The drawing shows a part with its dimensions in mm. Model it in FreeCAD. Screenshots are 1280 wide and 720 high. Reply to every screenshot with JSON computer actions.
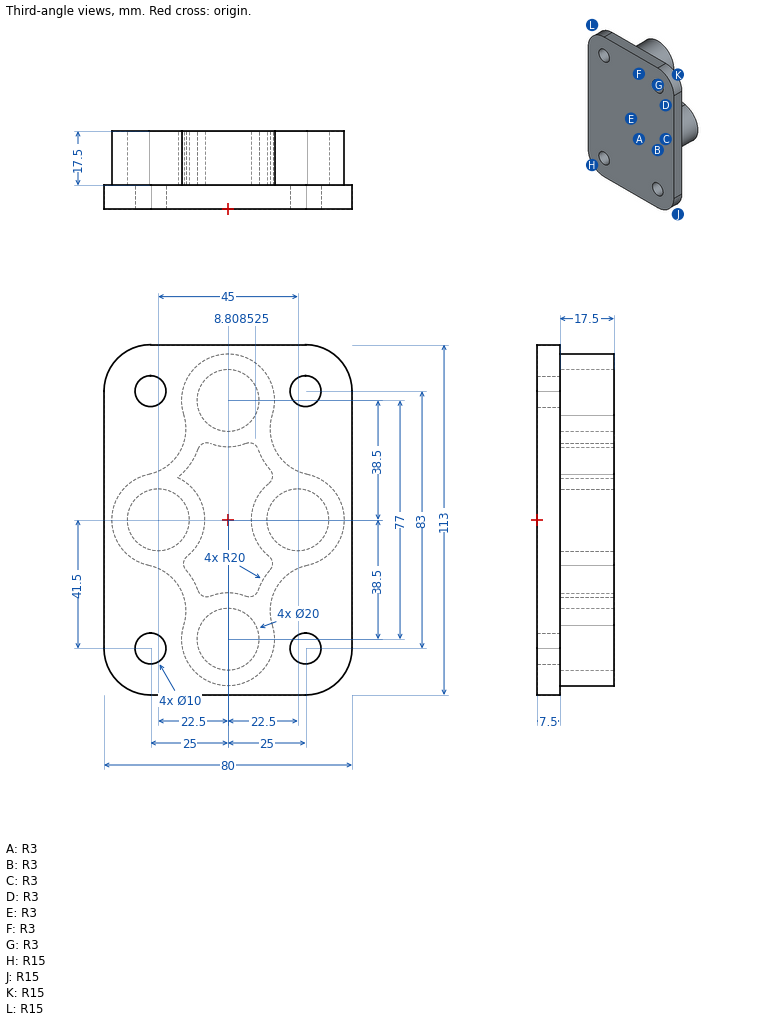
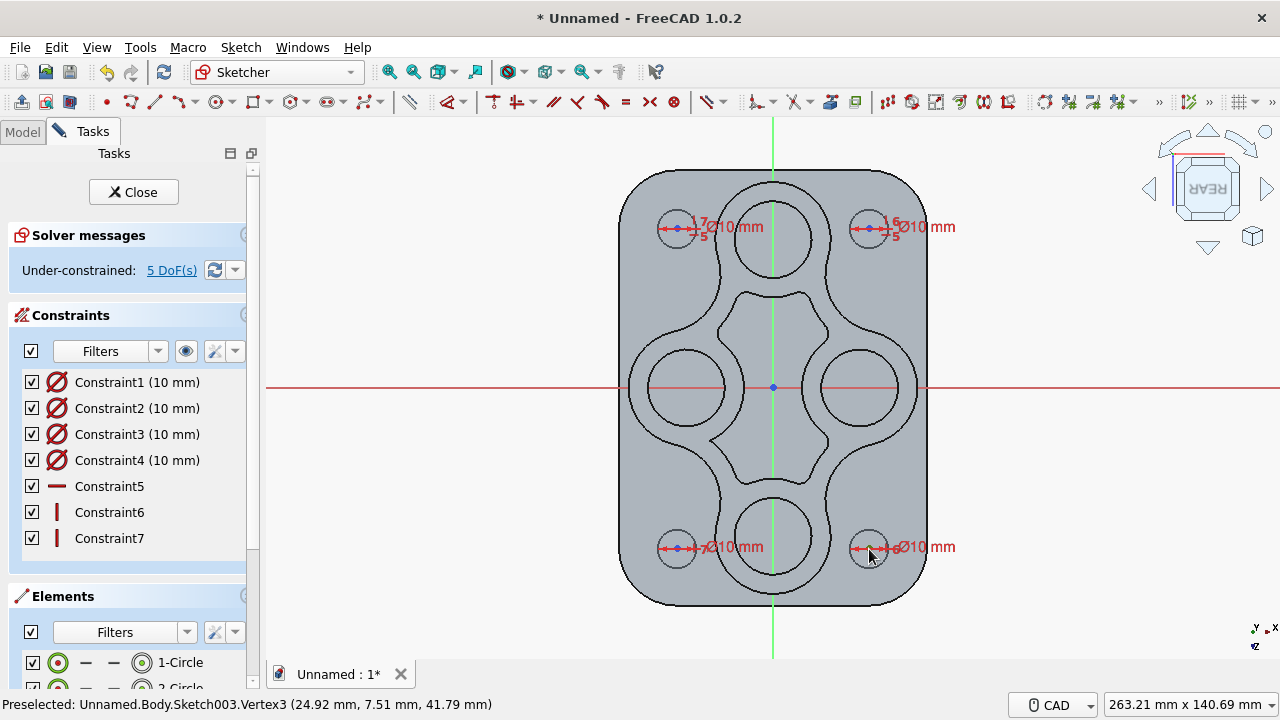
{"action": "left_click", "coordinate": [677, 549]}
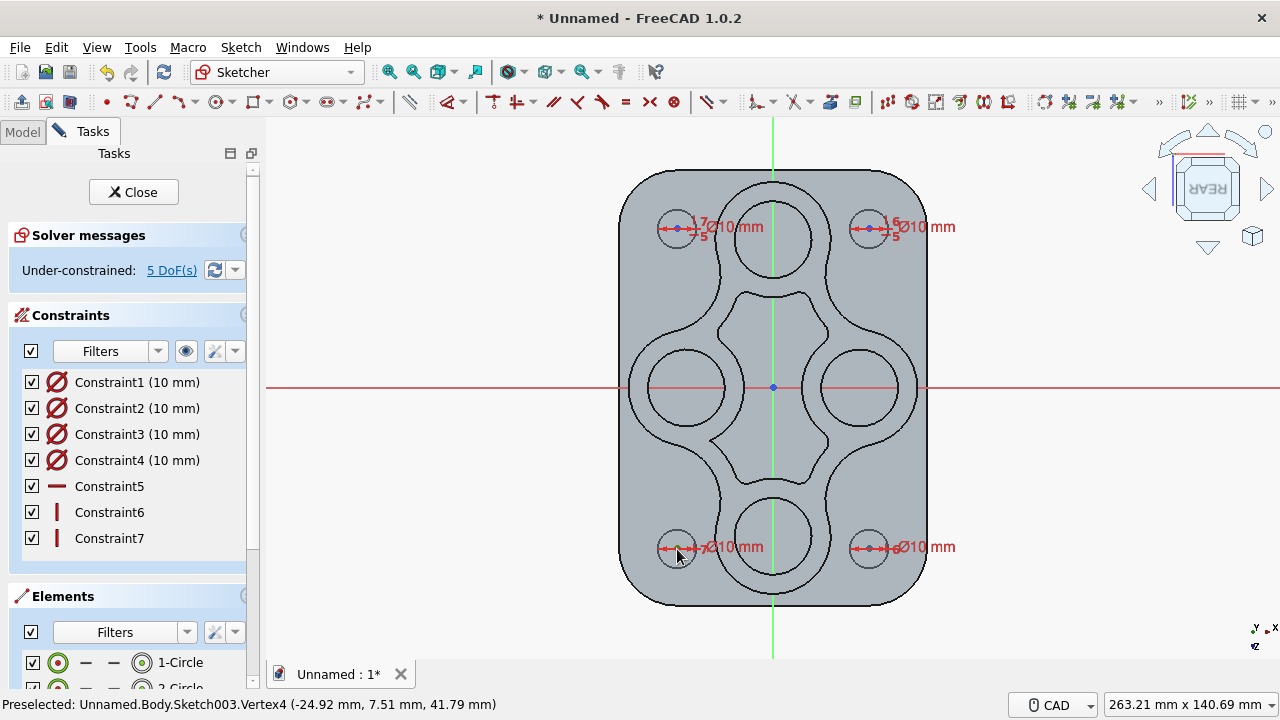
{"action": "left_click", "coordinate": [536, 102]}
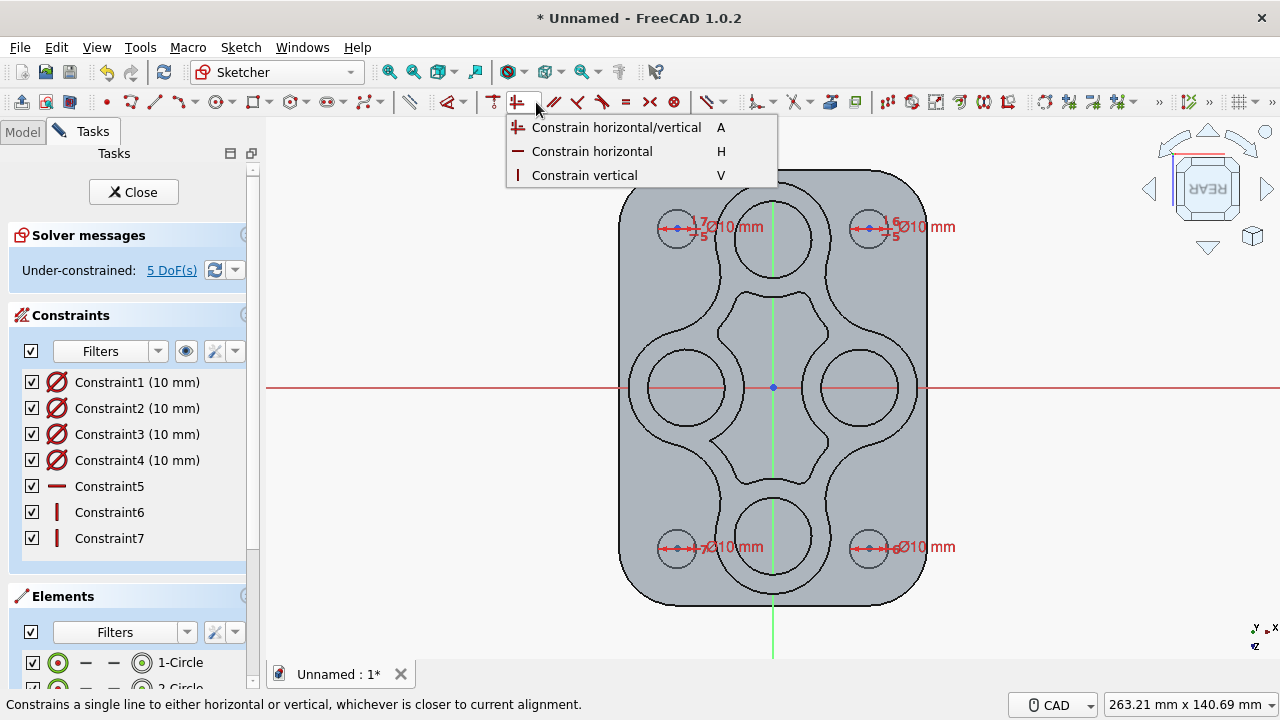
{"action": "left_click", "coordinate": [642, 151]}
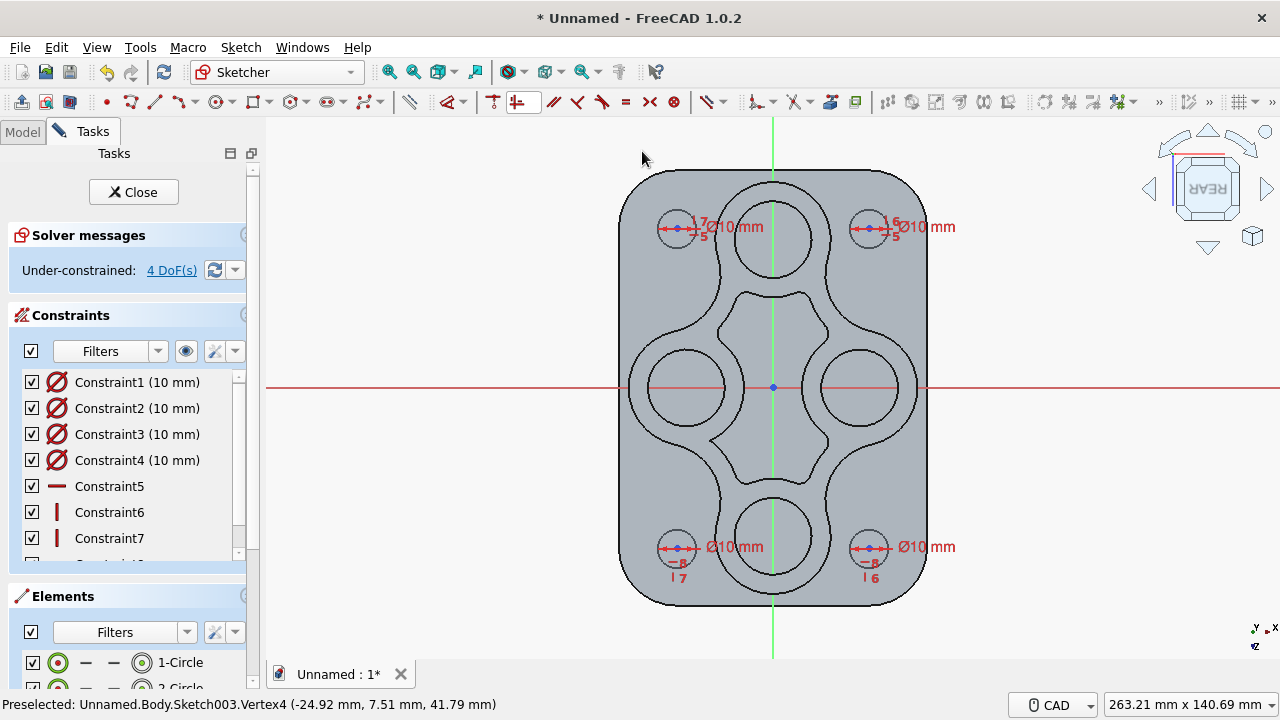
{"action": "key", "text": "d"}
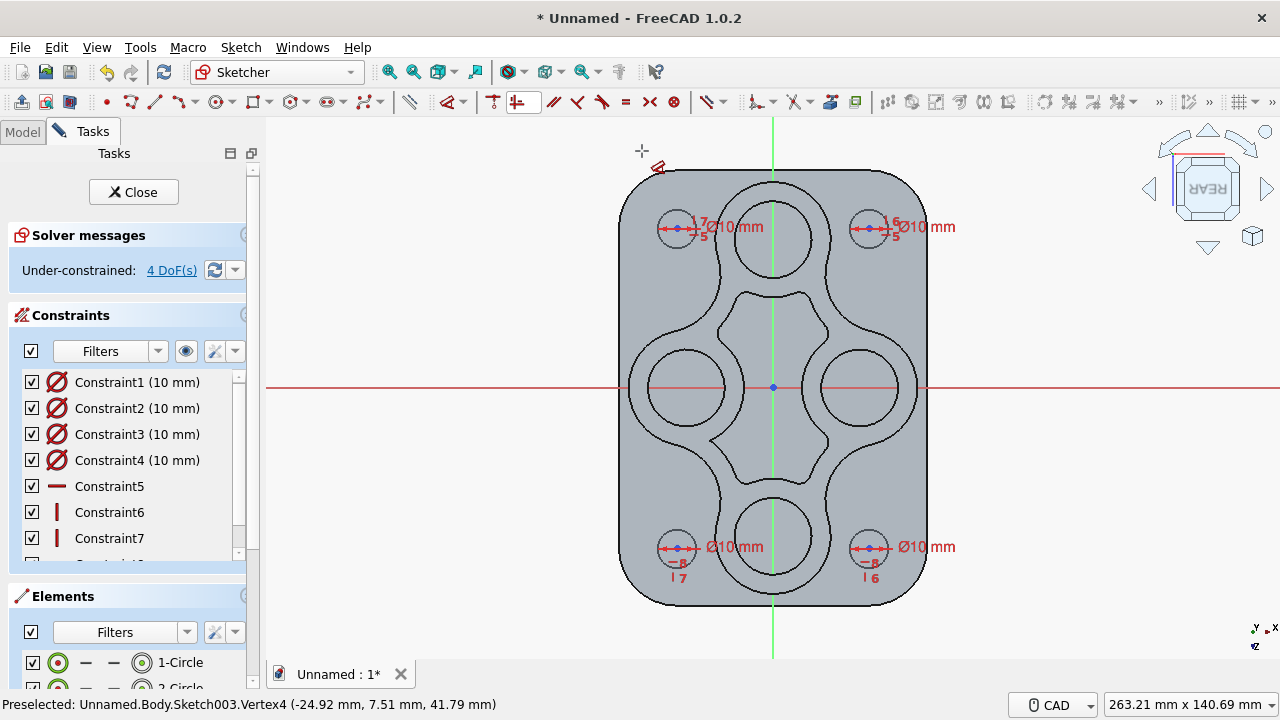
{"action": "left_click", "coordinate": [677, 229]}
{"action": "left_click", "coordinate": [725, 195]}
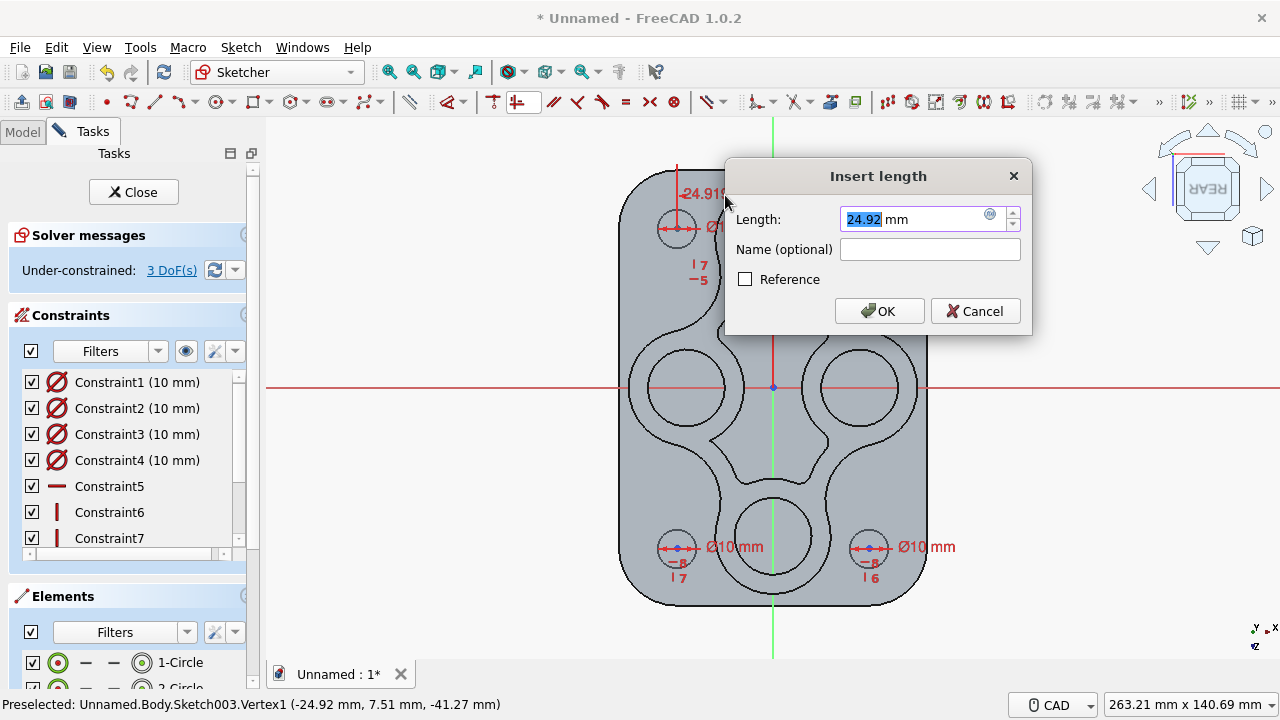
{"action": "type", "text": "25"}
{"action": "key", "text": "Return"}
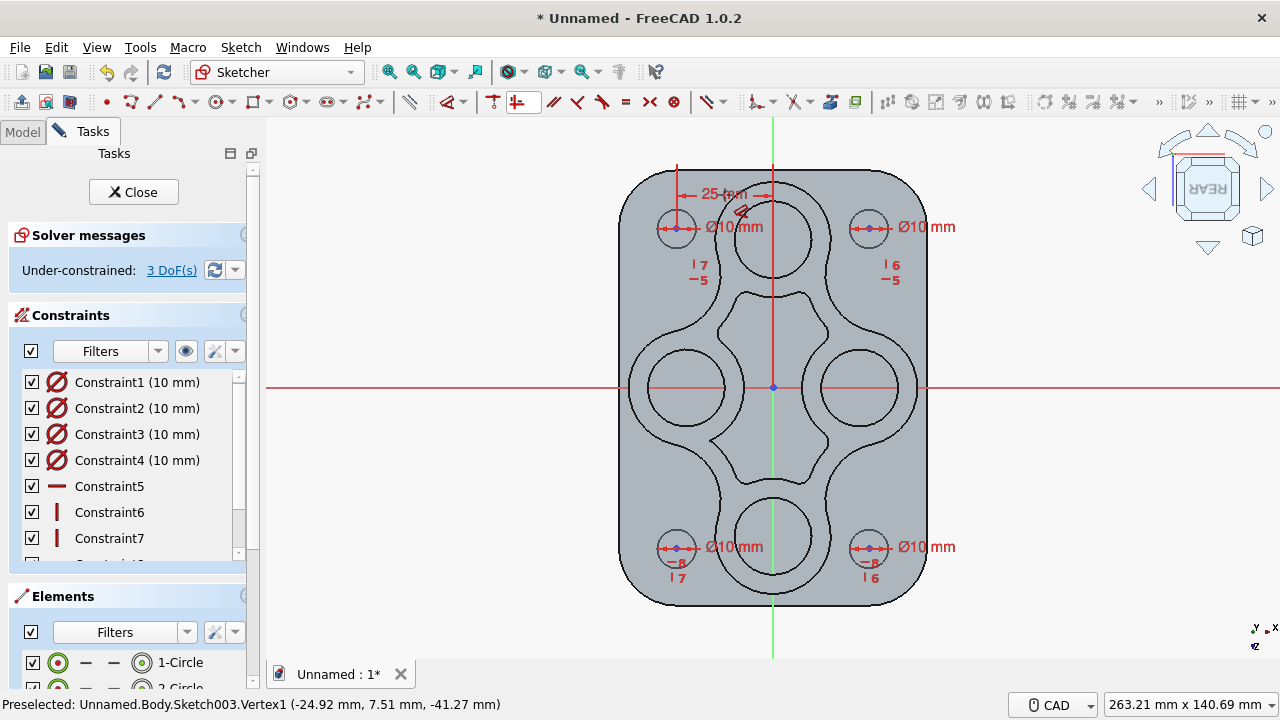
{"action": "left_click", "coordinate": [869, 229]}
{"action": "left_click", "coordinate": [821, 195]}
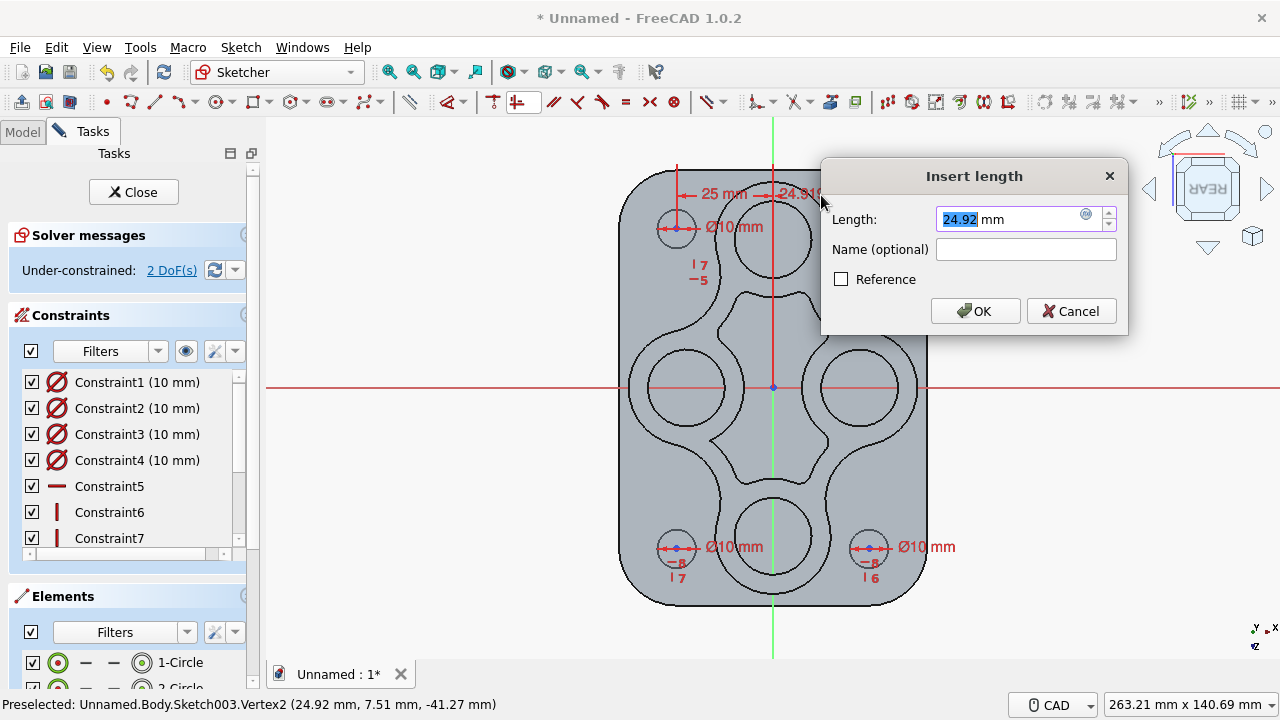
{"action": "type", "text": "25"}
{"action": "key", "text": "Return"}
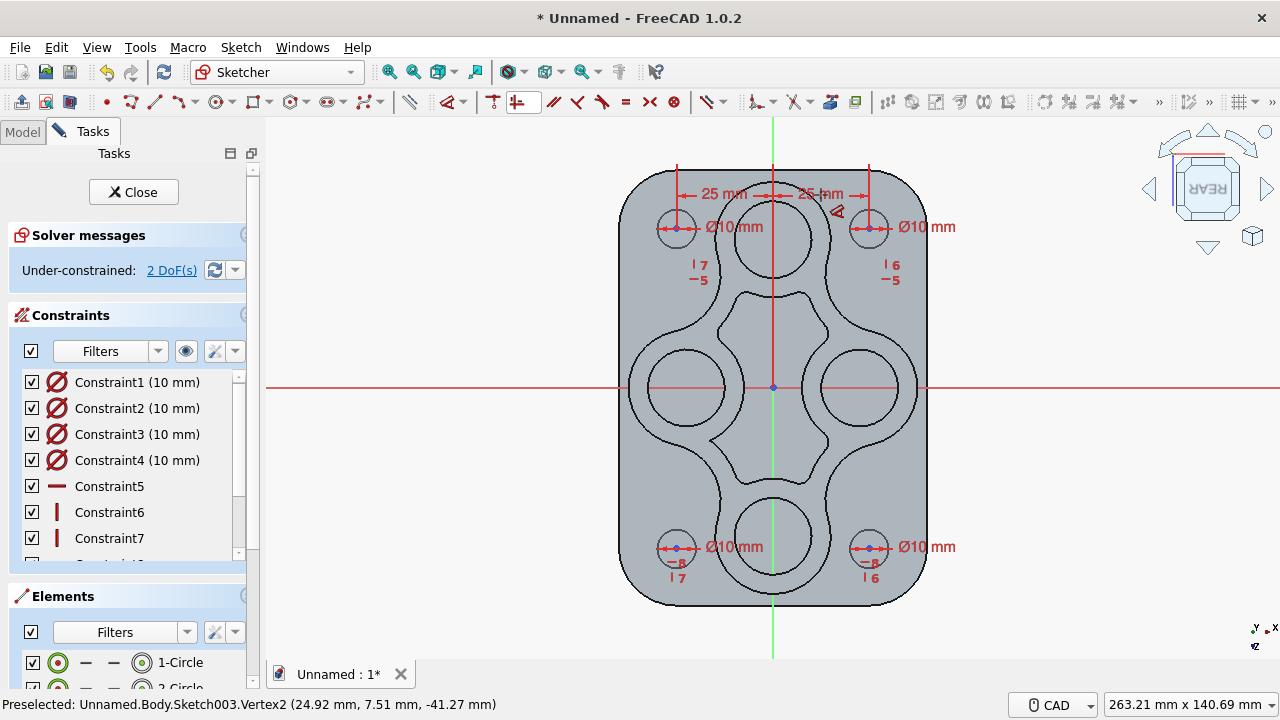
{"action": "left_click", "coordinate": [869, 229]}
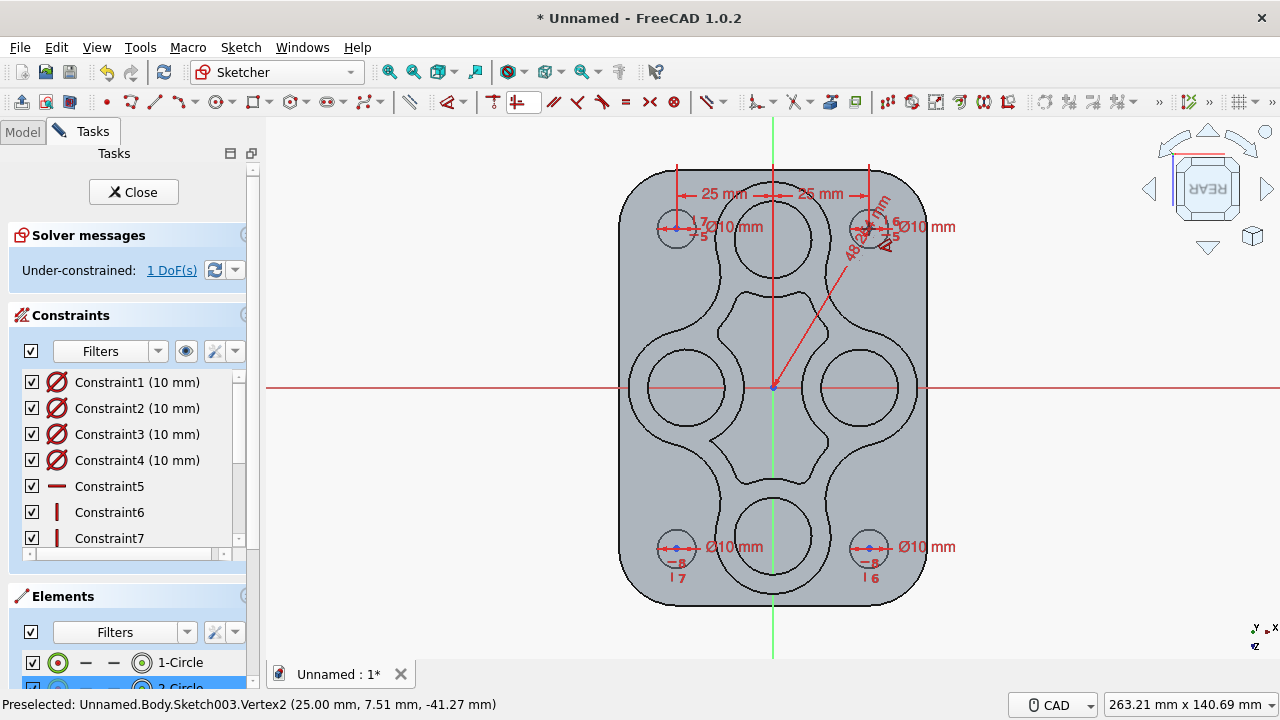
{"action": "left_click", "coordinate": [869, 549]}
{"action": "left_click", "coordinate": [903, 315]}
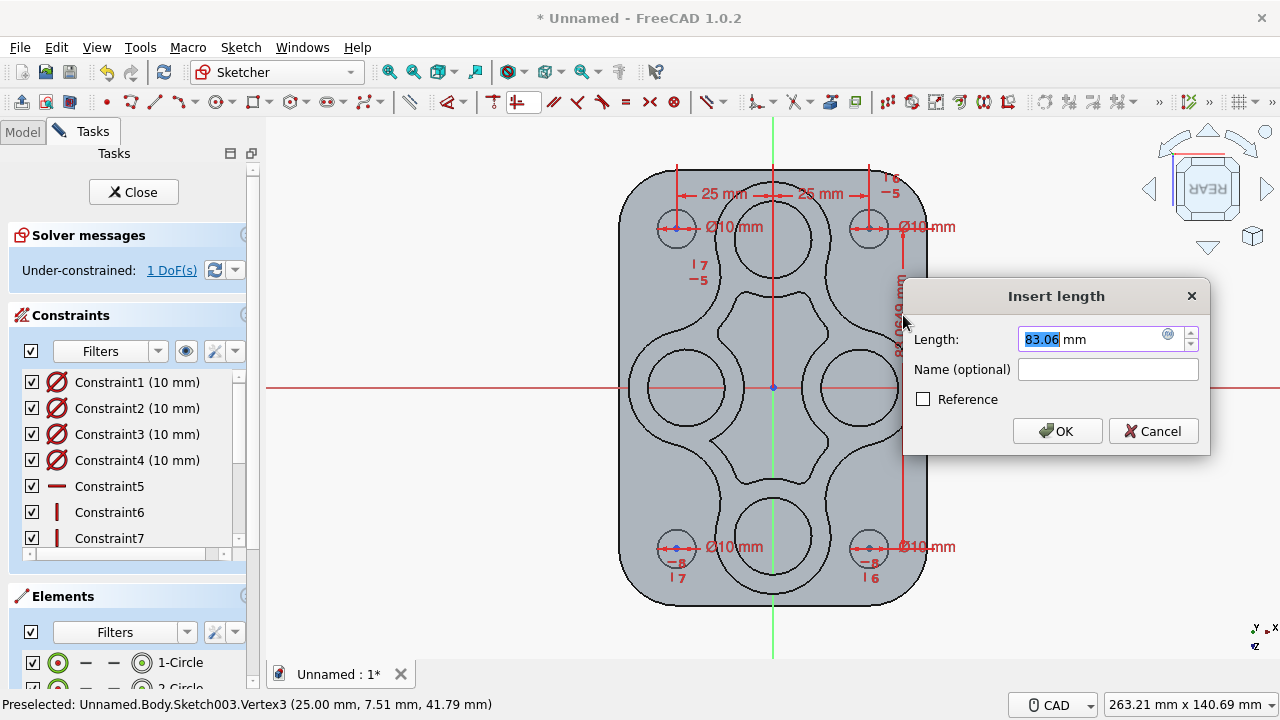
{"action": "type", "text": "83"}
{"action": "key", "text": "Return"}